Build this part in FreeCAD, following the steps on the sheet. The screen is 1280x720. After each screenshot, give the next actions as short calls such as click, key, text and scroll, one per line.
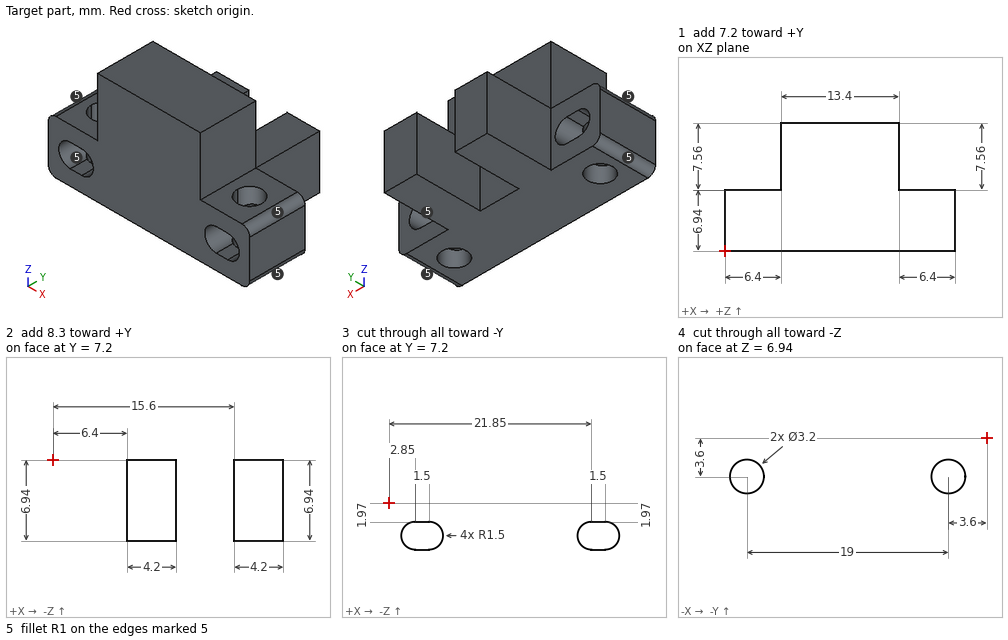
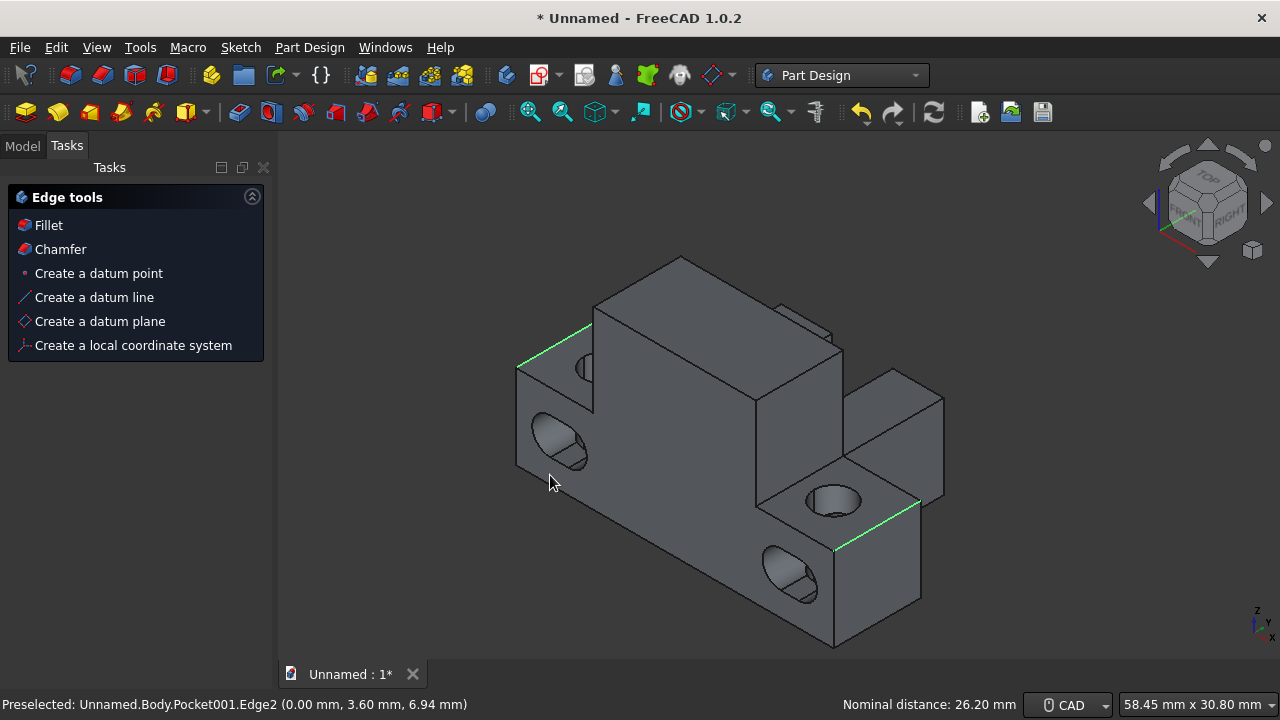
key(1)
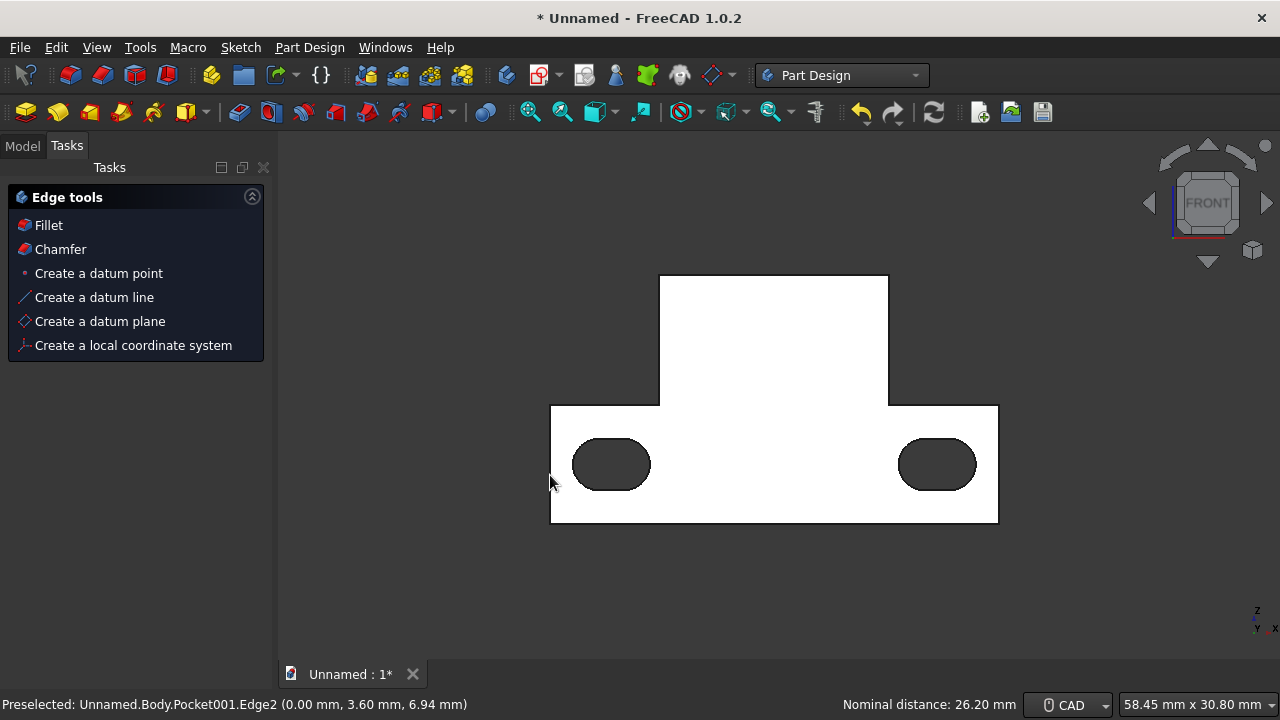
key(3)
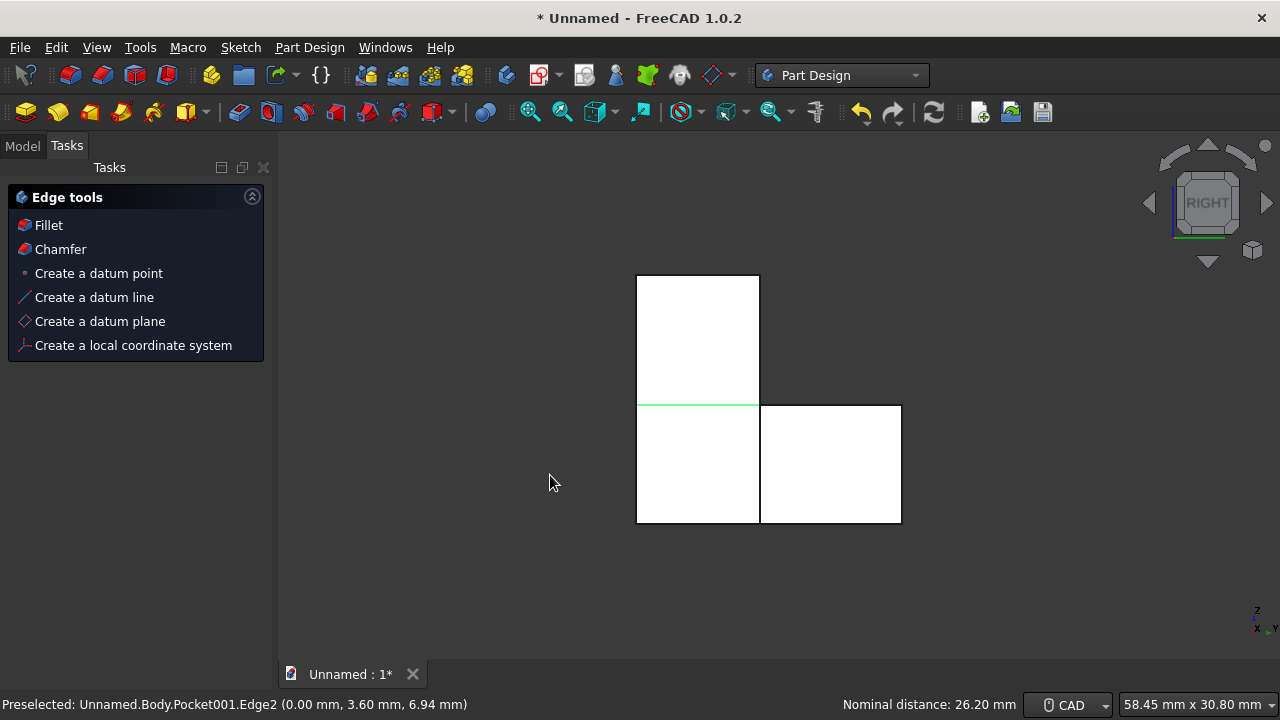
click(698, 523, ctrl)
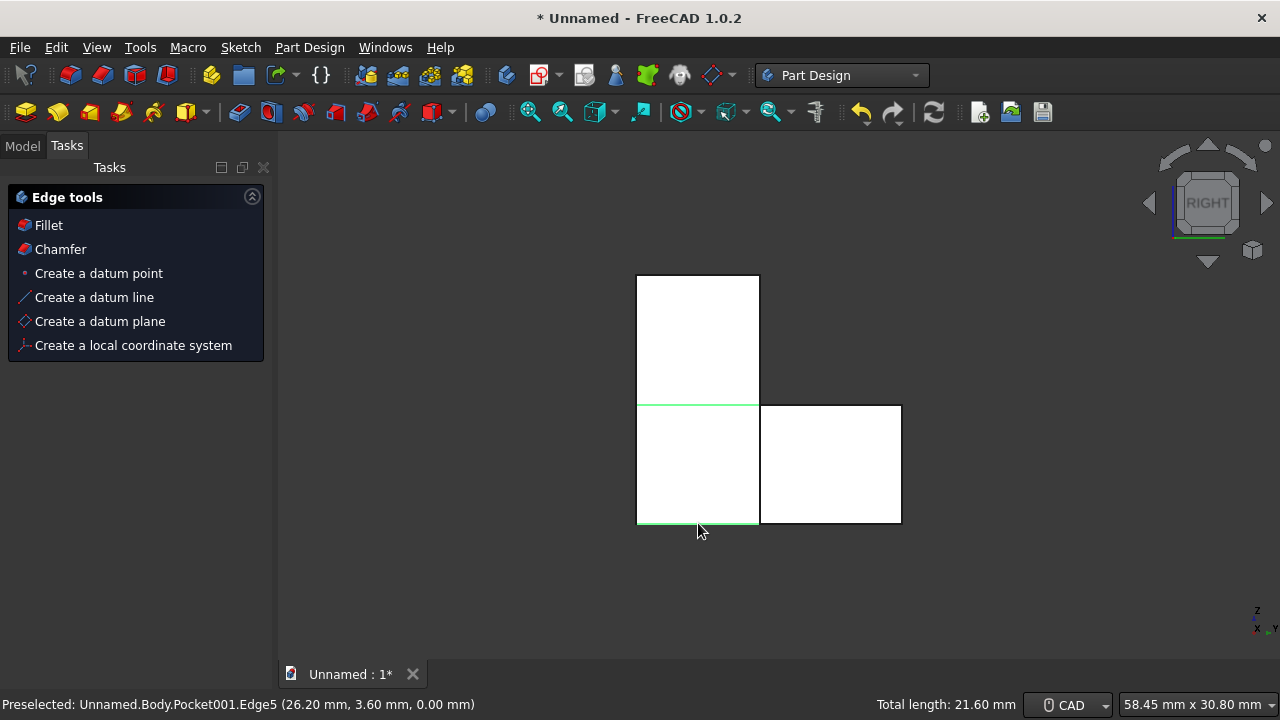
key(5)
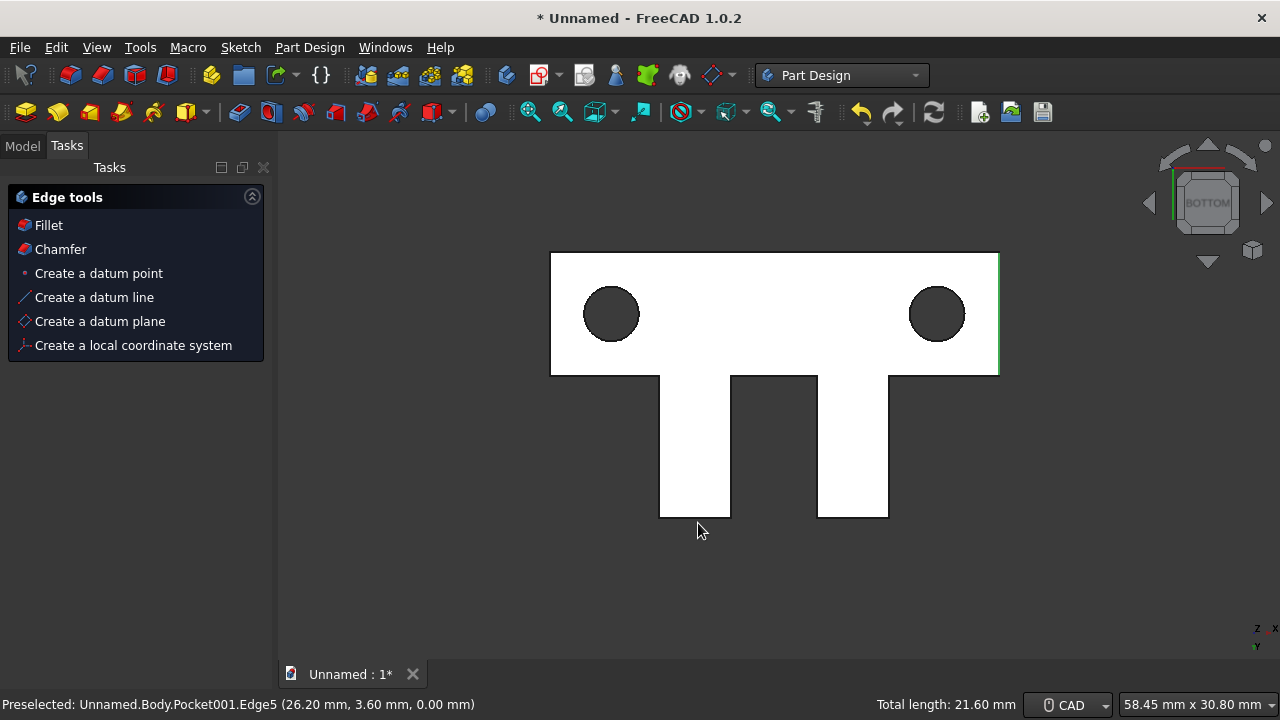
key(4)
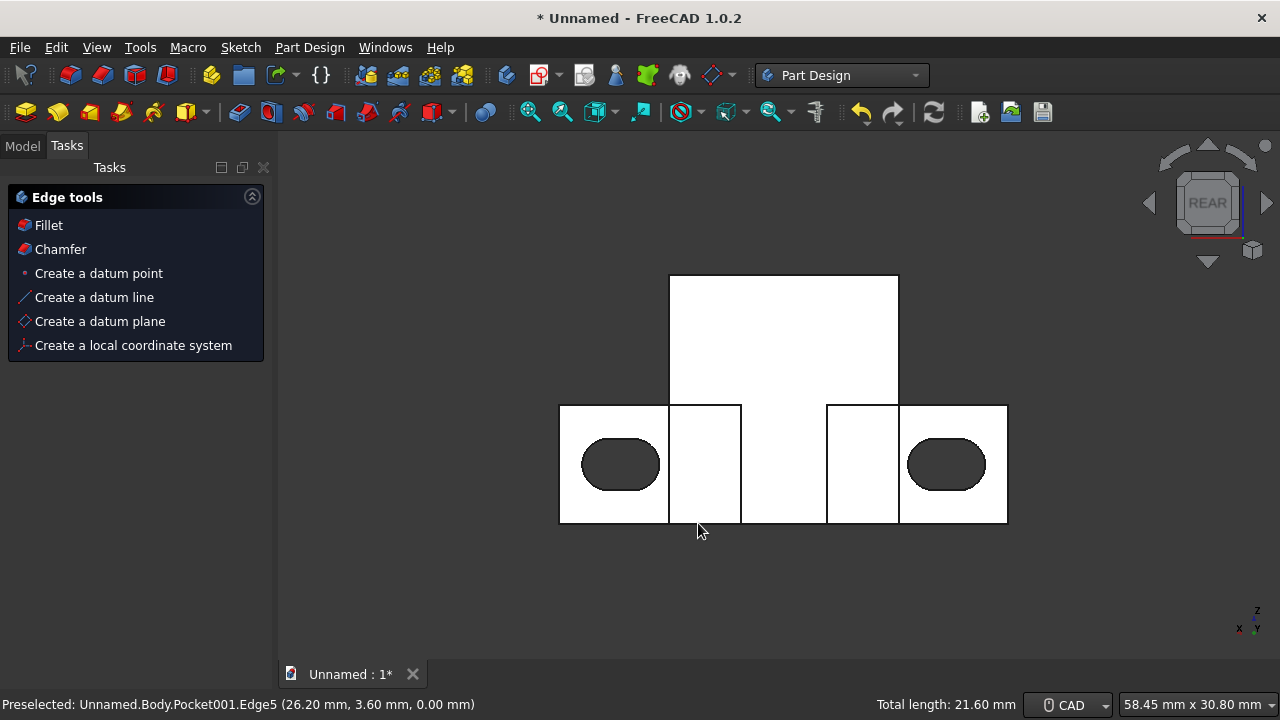
key(6)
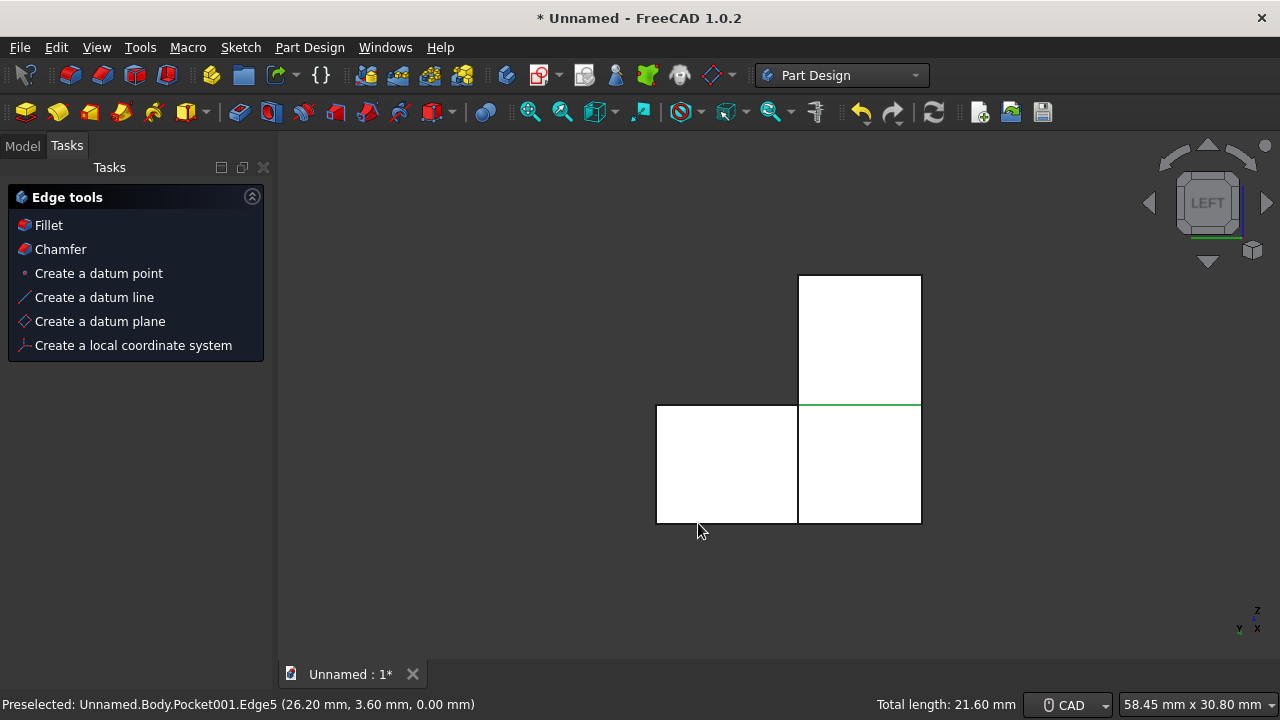
click(860, 523, ctrl)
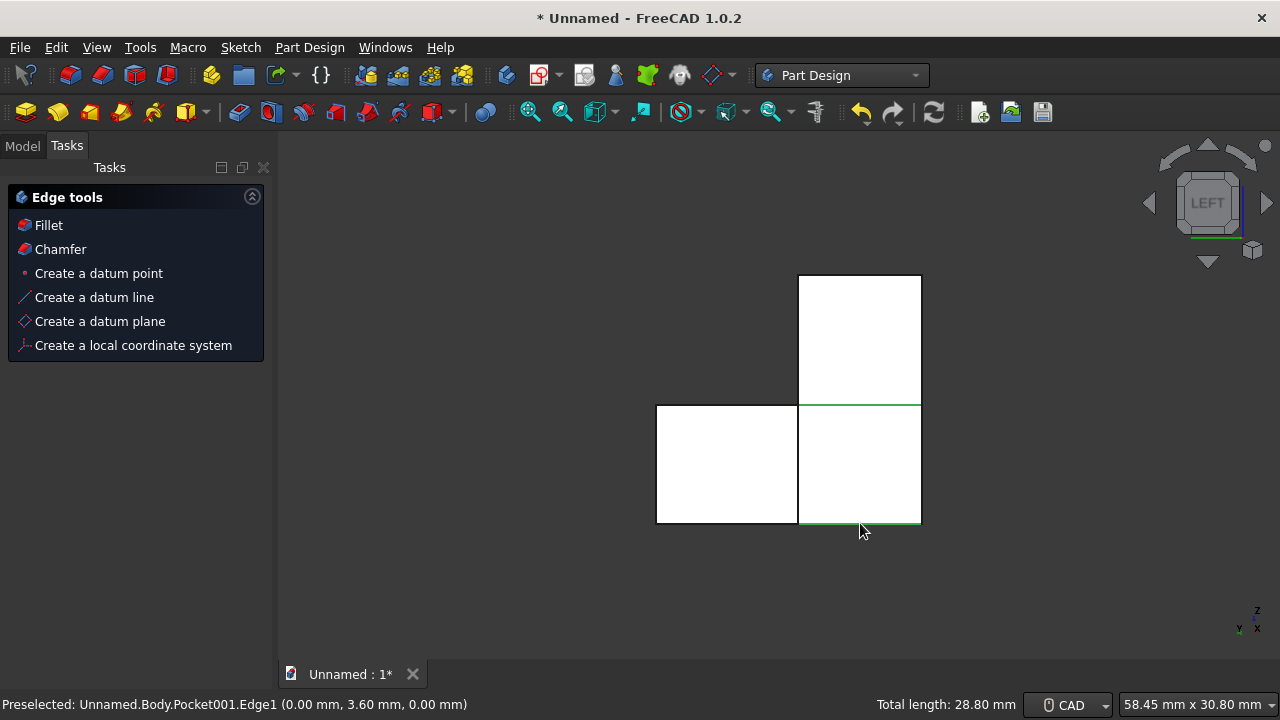
click(72, 76)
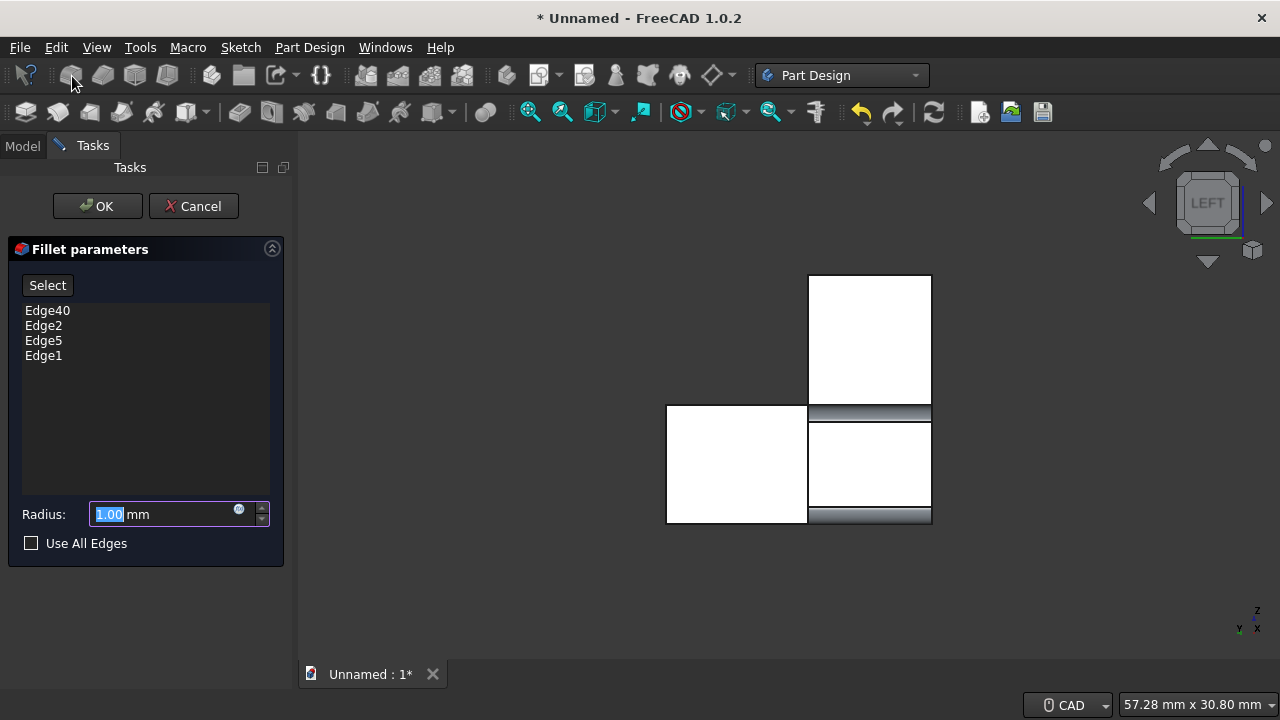
text(1)
key(Tab)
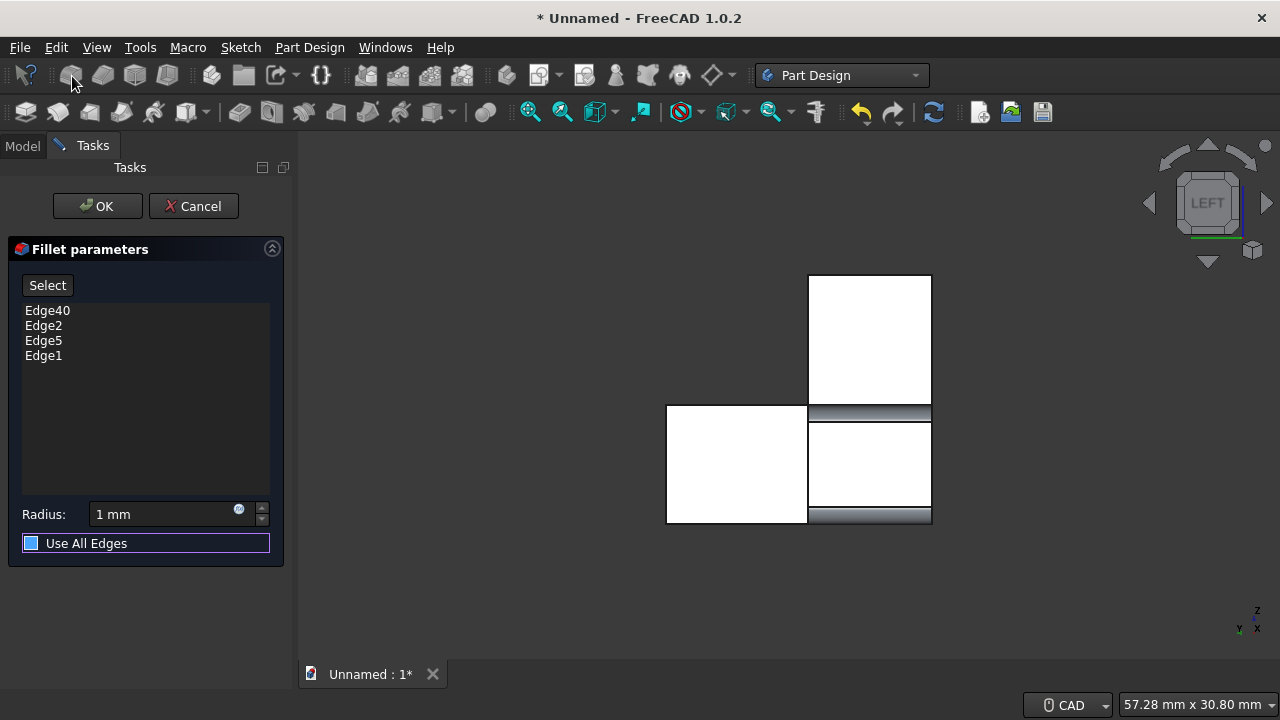
click(98, 206)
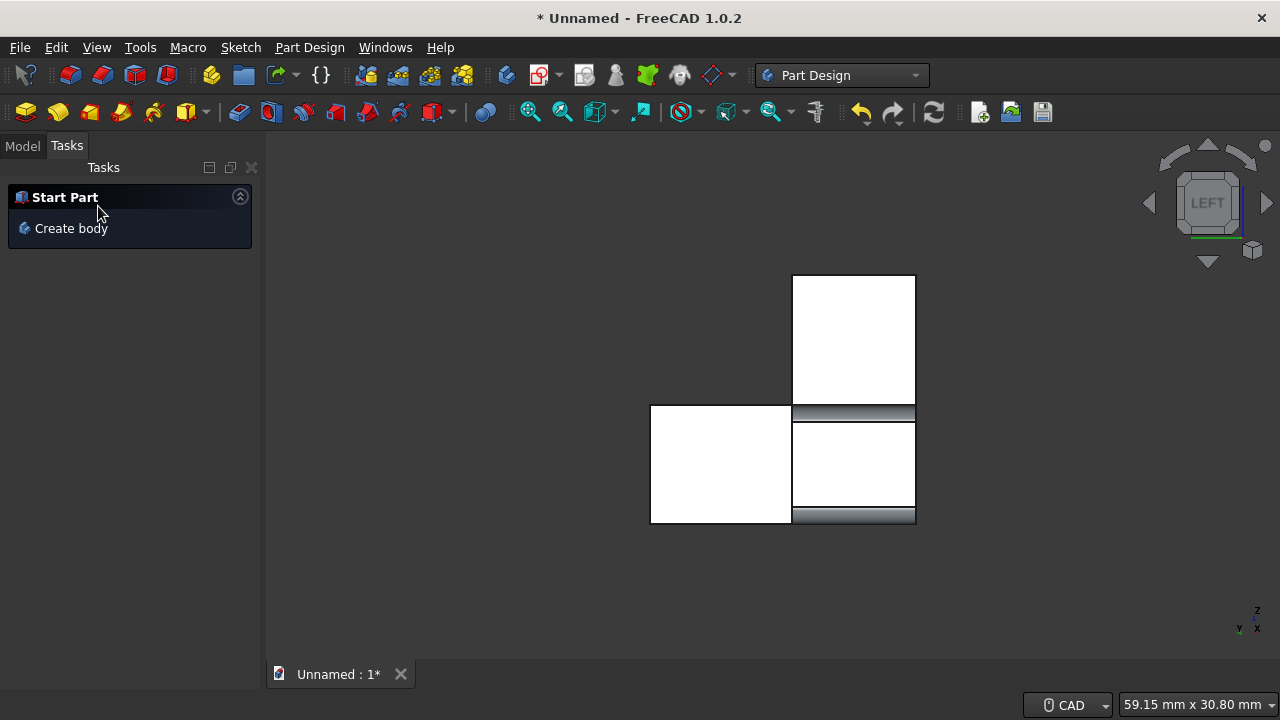
key(0)